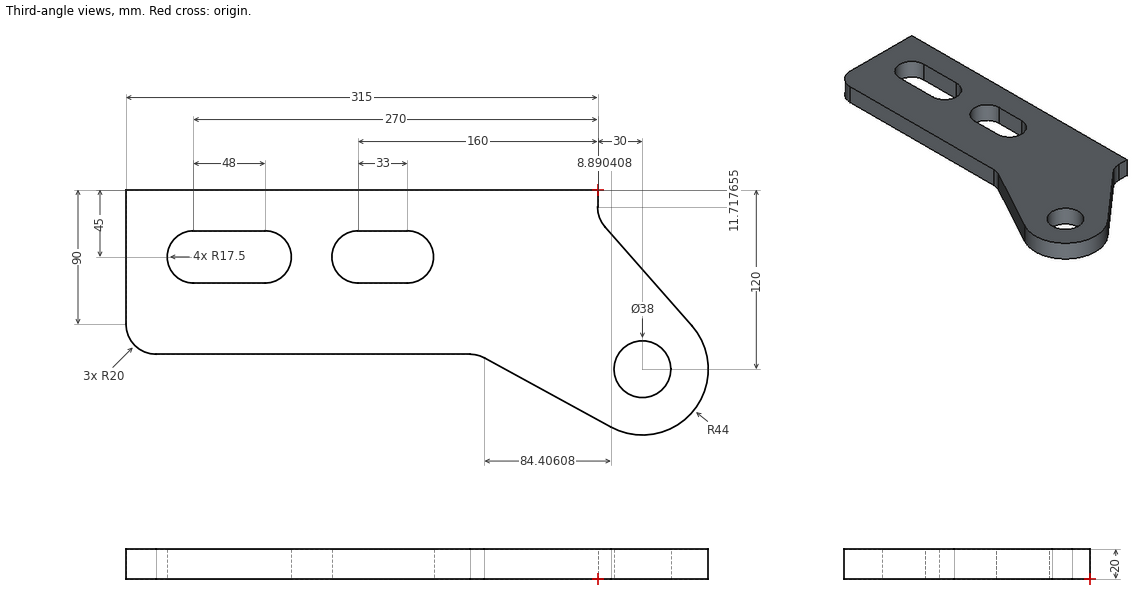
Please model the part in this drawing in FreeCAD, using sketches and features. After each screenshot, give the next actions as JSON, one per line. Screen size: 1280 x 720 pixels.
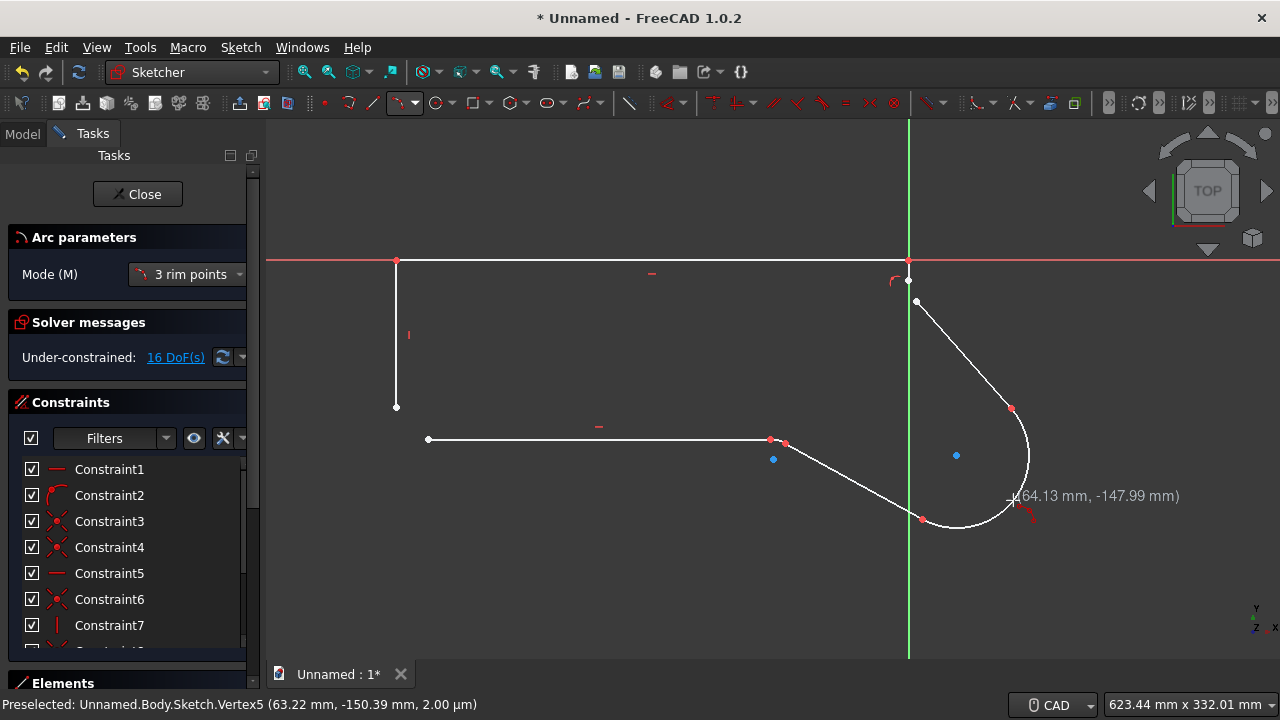
{"action": "scroll", "coordinate": [917, 301], "scroll_direction": "up", "scroll_amount": 4}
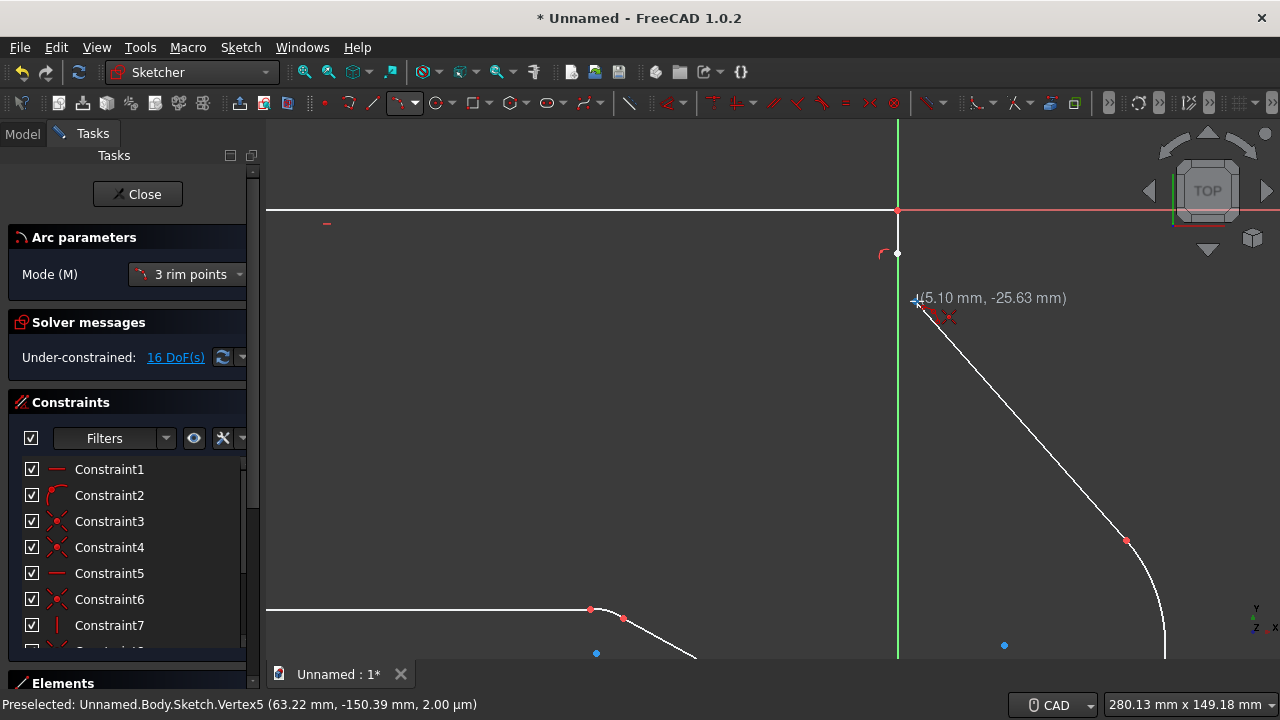
{"action": "left_click", "coordinate": [916, 302]}
{"action": "left_click", "coordinate": [898, 254]}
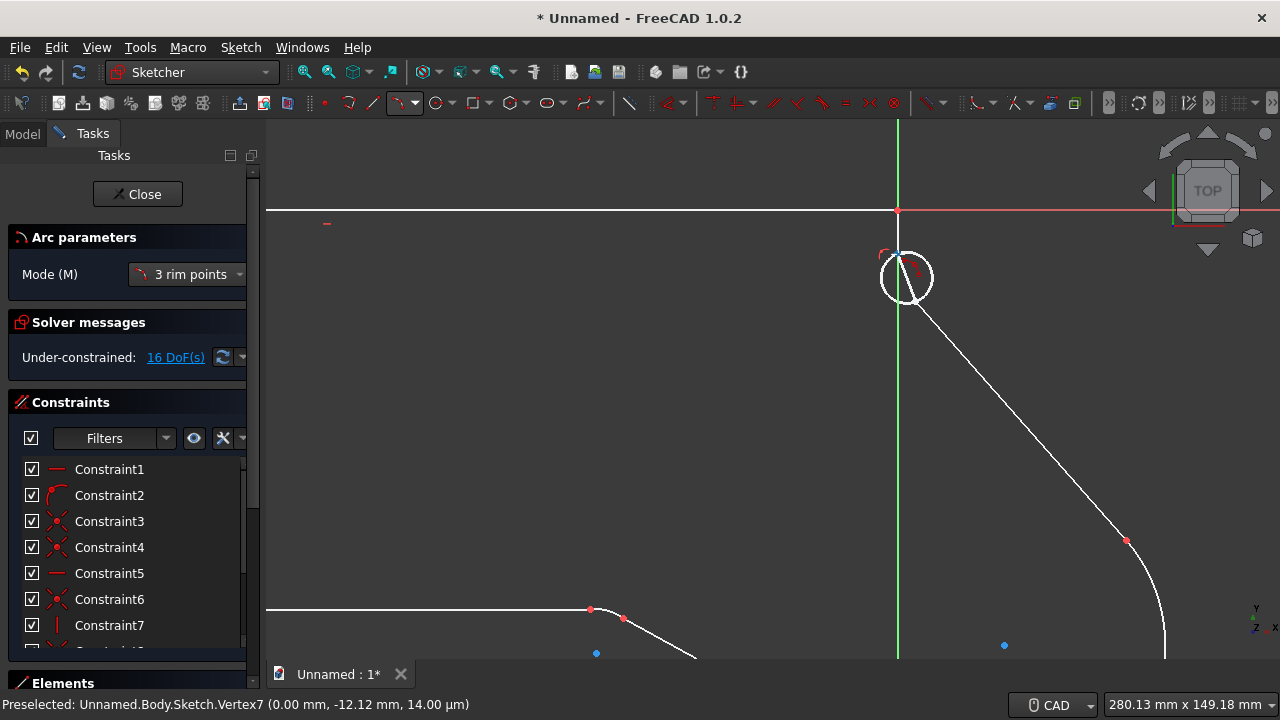
{"action": "scroll", "coordinate": [902, 278], "scroll_direction": "up", "scroll_amount": 7}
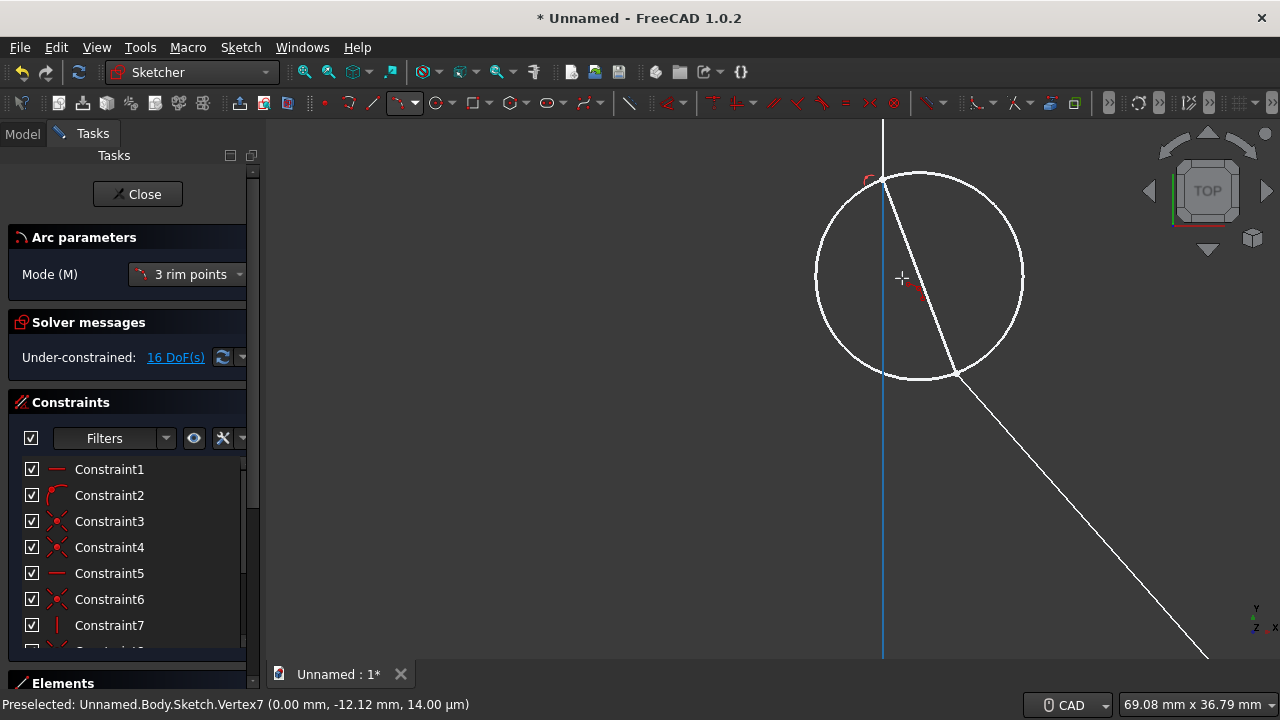
{"action": "left_click", "coordinate": [902, 277]}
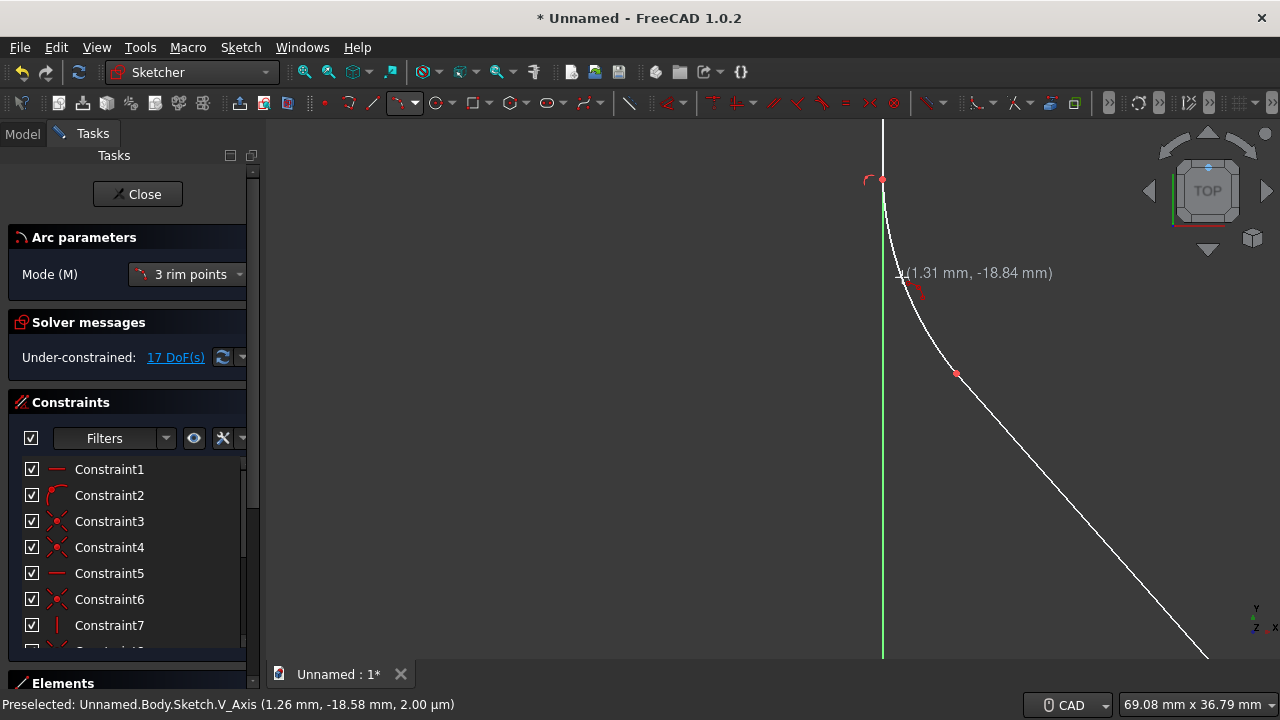
{"action": "scroll", "coordinate": [912, 292], "scroll_direction": "down", "scroll_amount": 11}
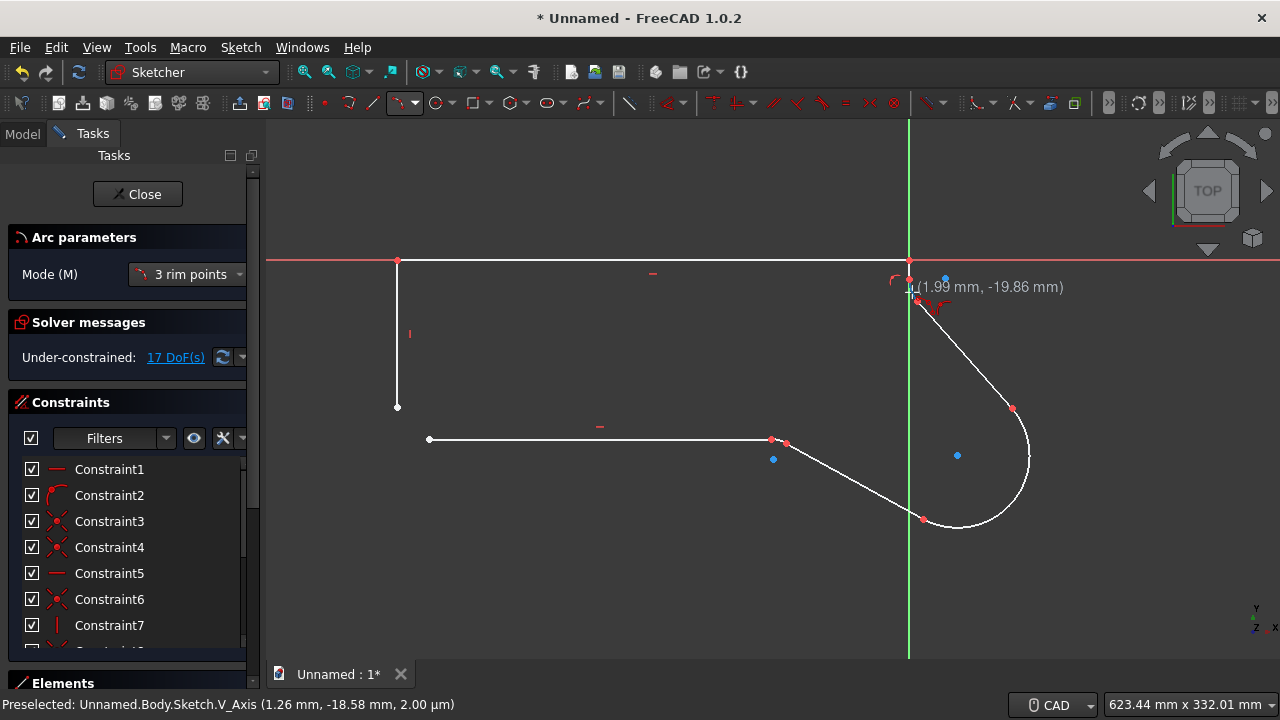
{"action": "left_click", "coordinate": [397, 408]}
{"action": "left_click", "coordinate": [429, 440]}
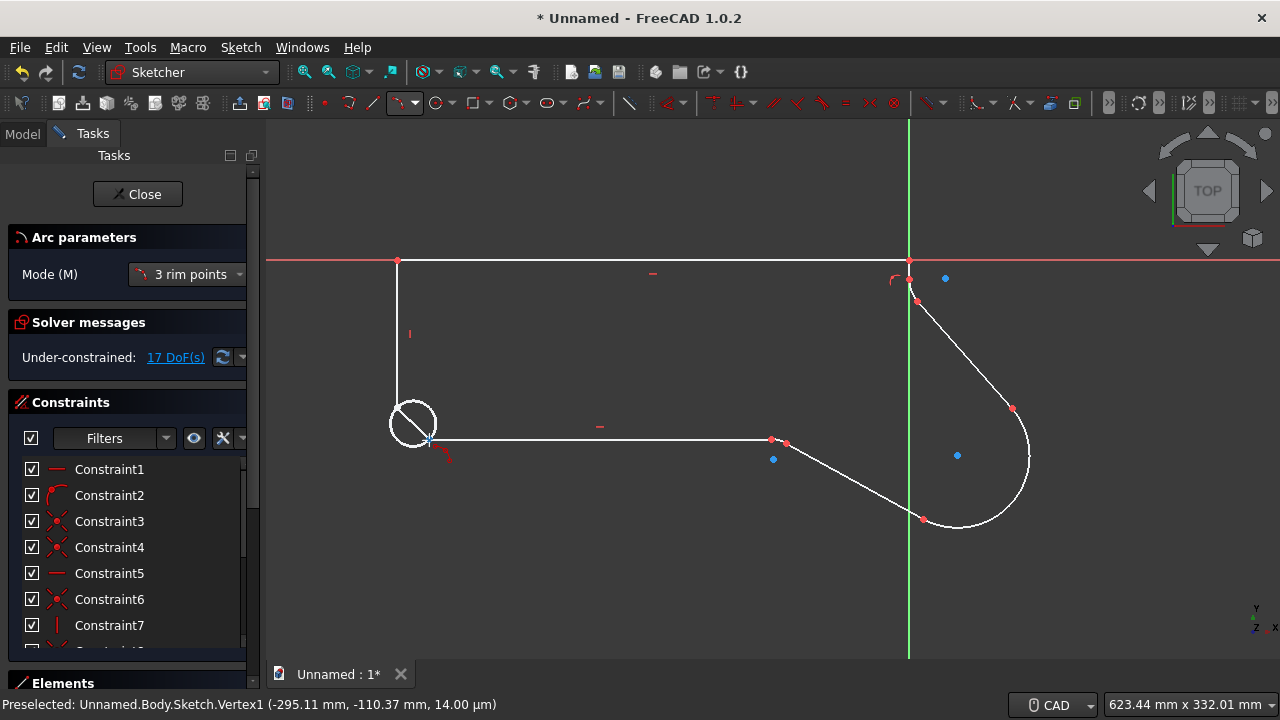
{"action": "scroll", "coordinate": [407, 429], "scroll_direction": "up", "scroll_amount": 3}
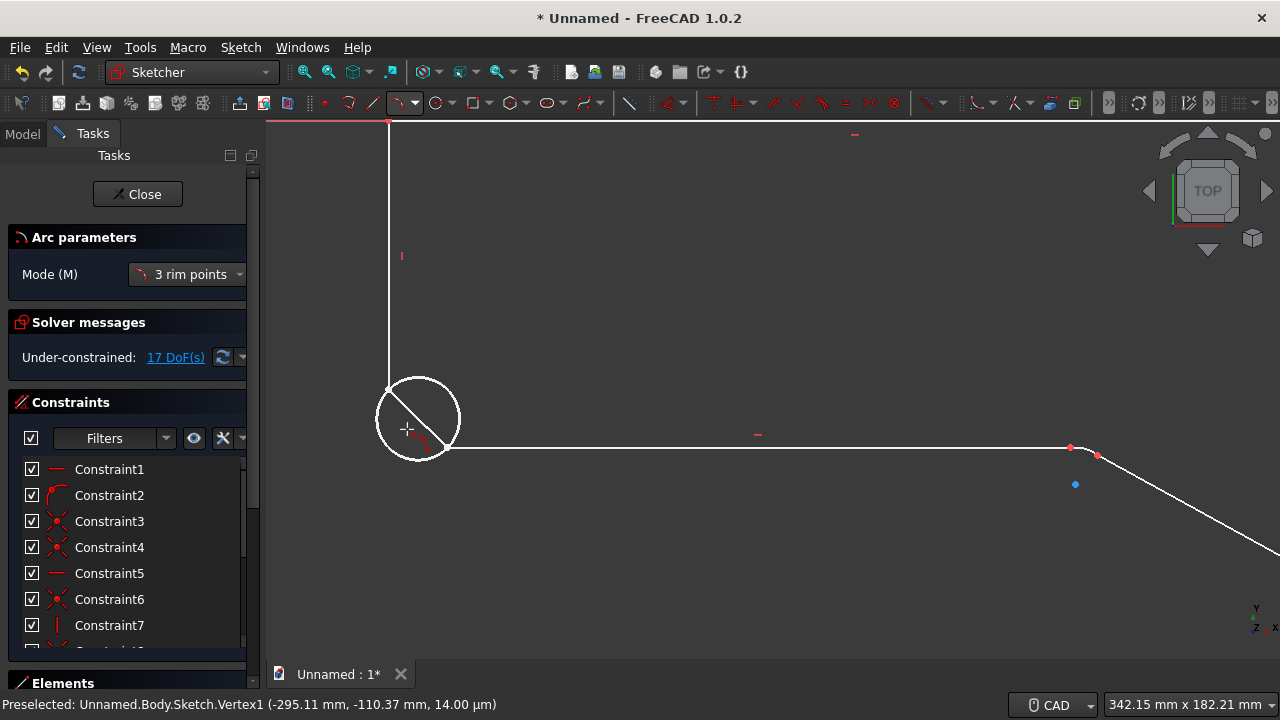
{"action": "left_click", "coordinate": [406, 429]}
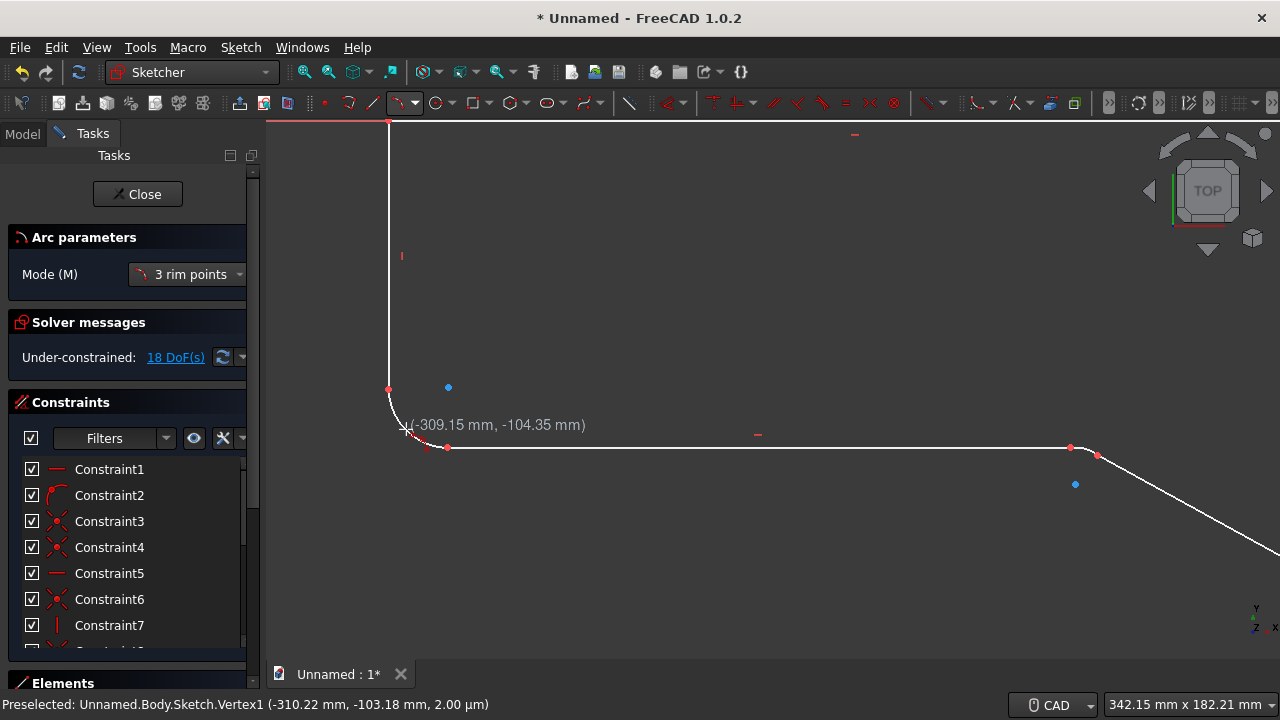
{"action": "left_click", "coordinate": [548, 104]}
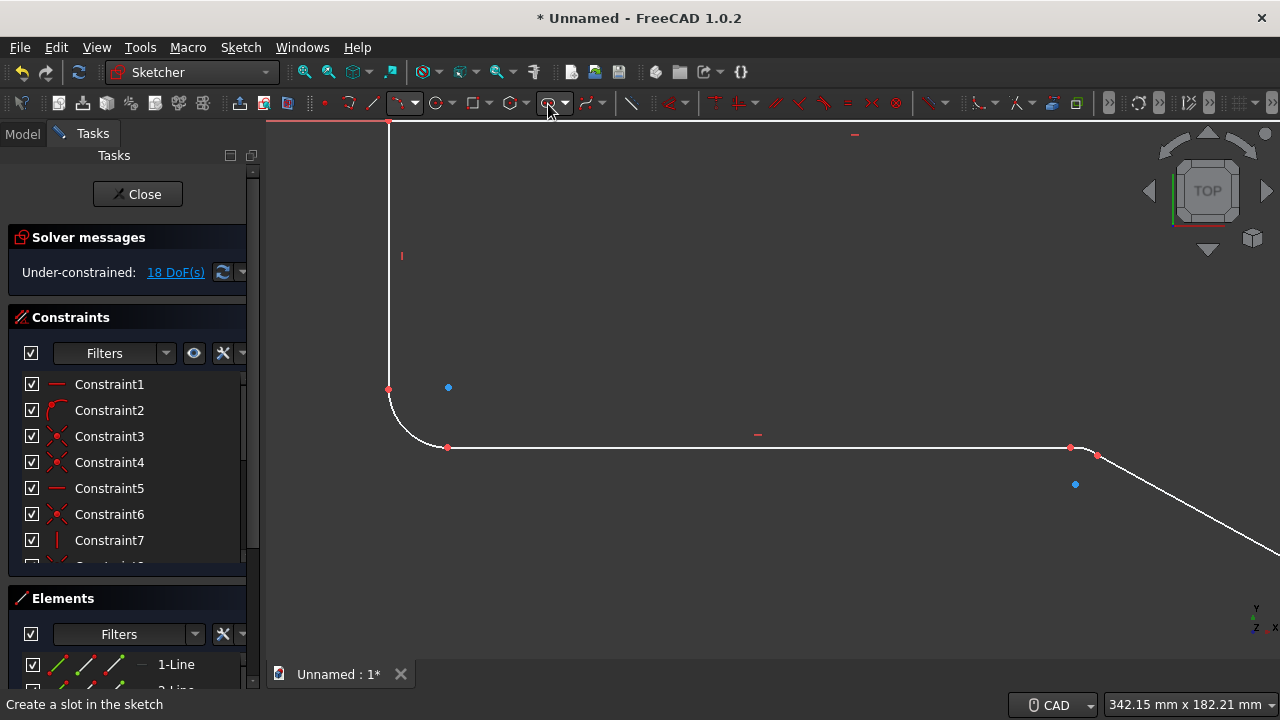
{"action": "left_click", "coordinate": [522, 254]}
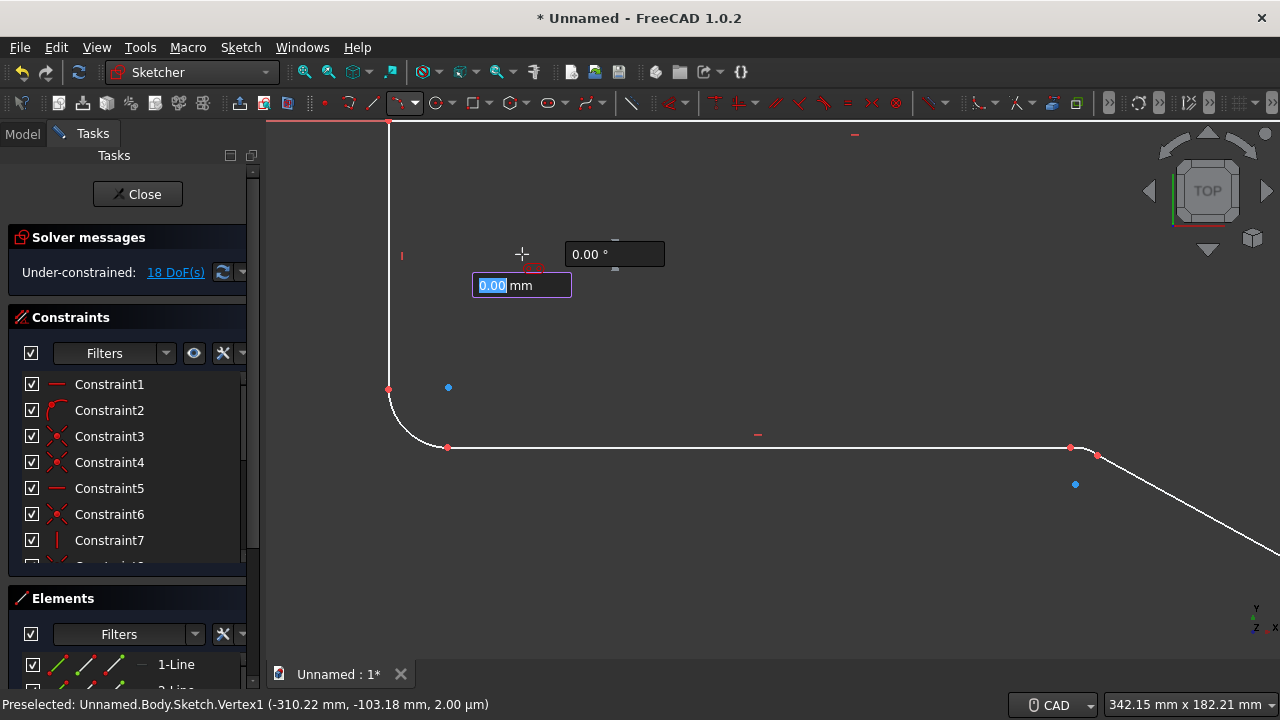
{"action": "left_click", "coordinate": [664, 254]}